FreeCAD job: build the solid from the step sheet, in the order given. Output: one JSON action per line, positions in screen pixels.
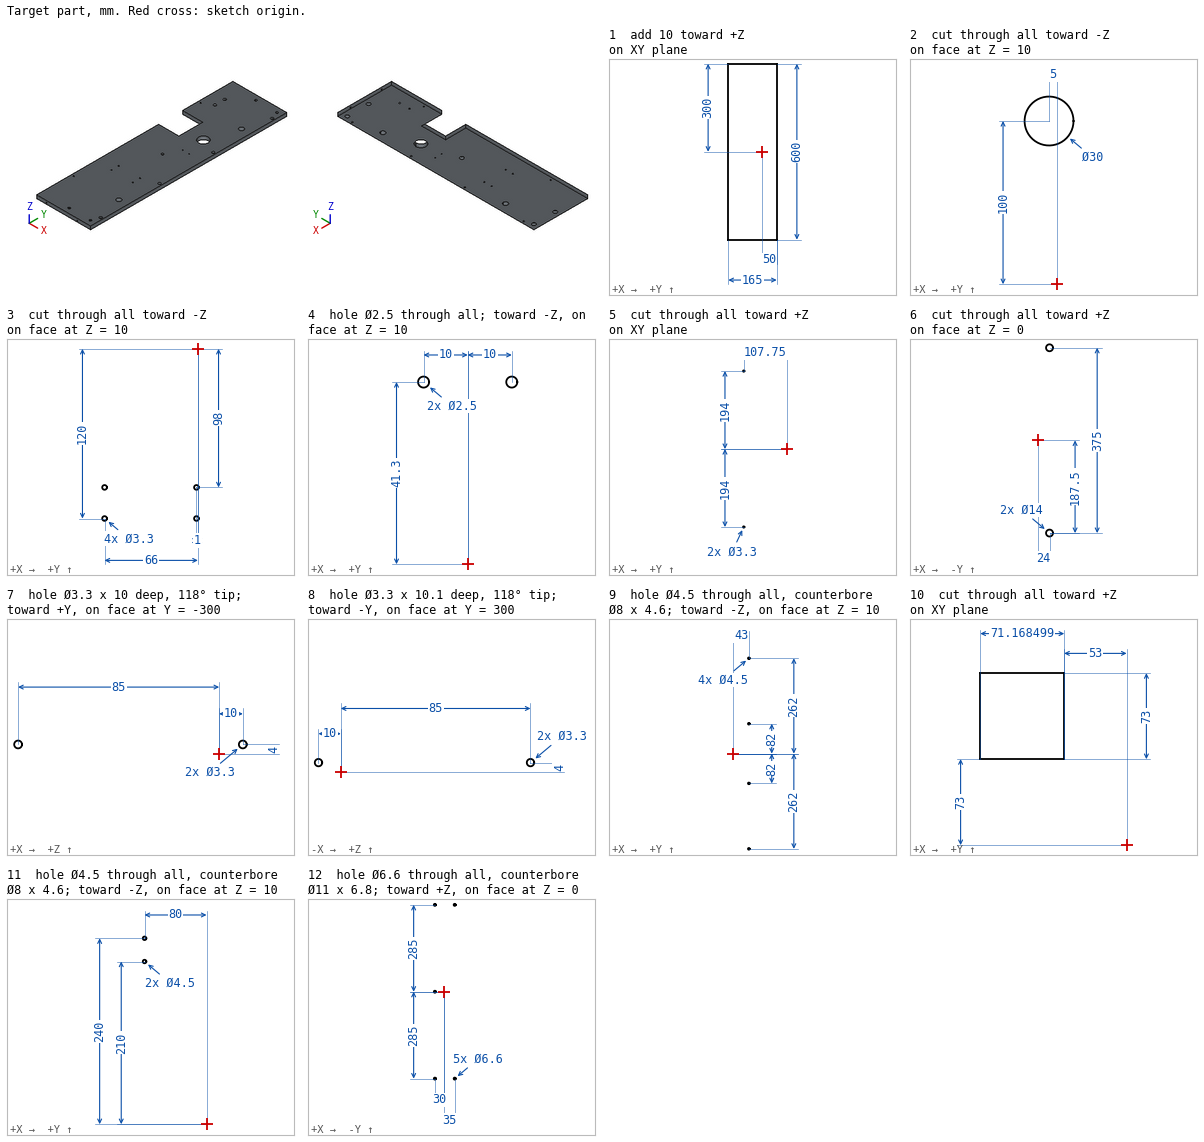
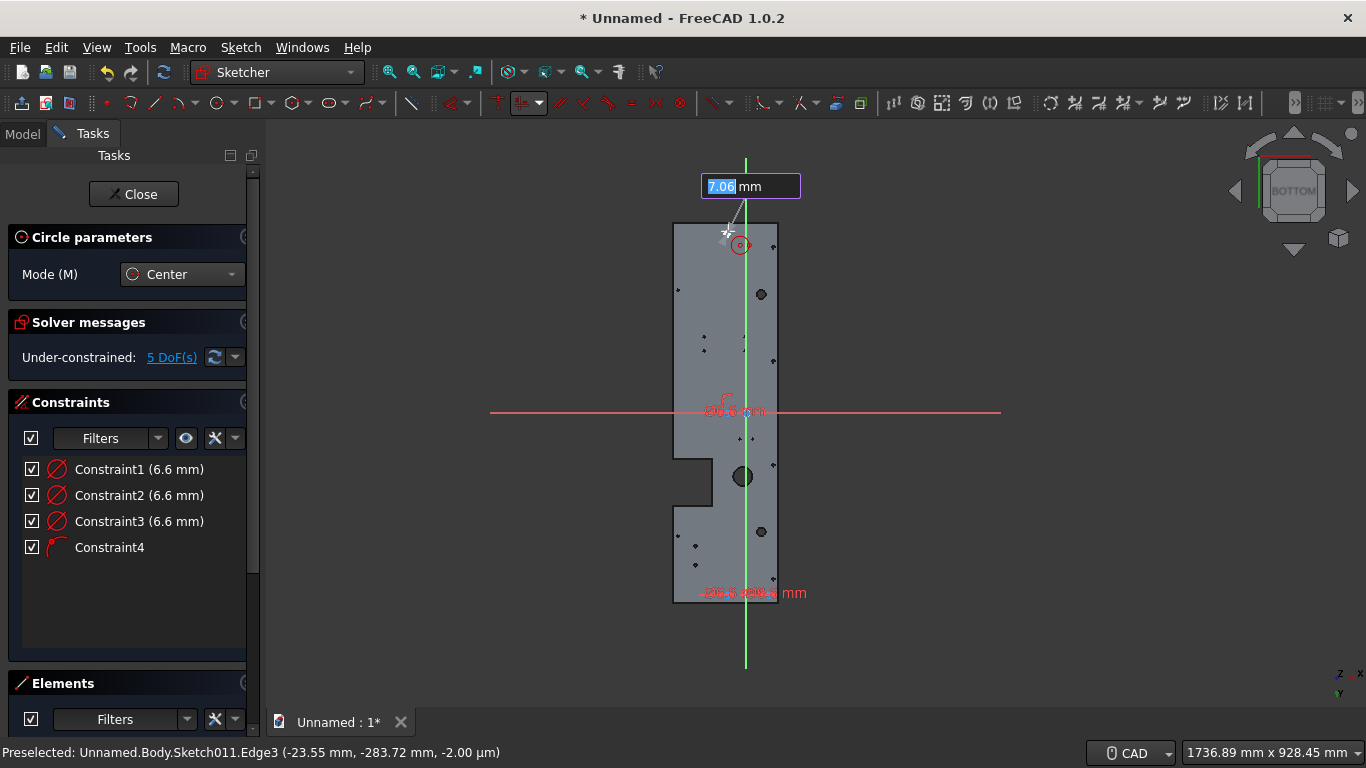
{"action": "type", "text": "6.6"}
{"action": "key", "text": "Return"}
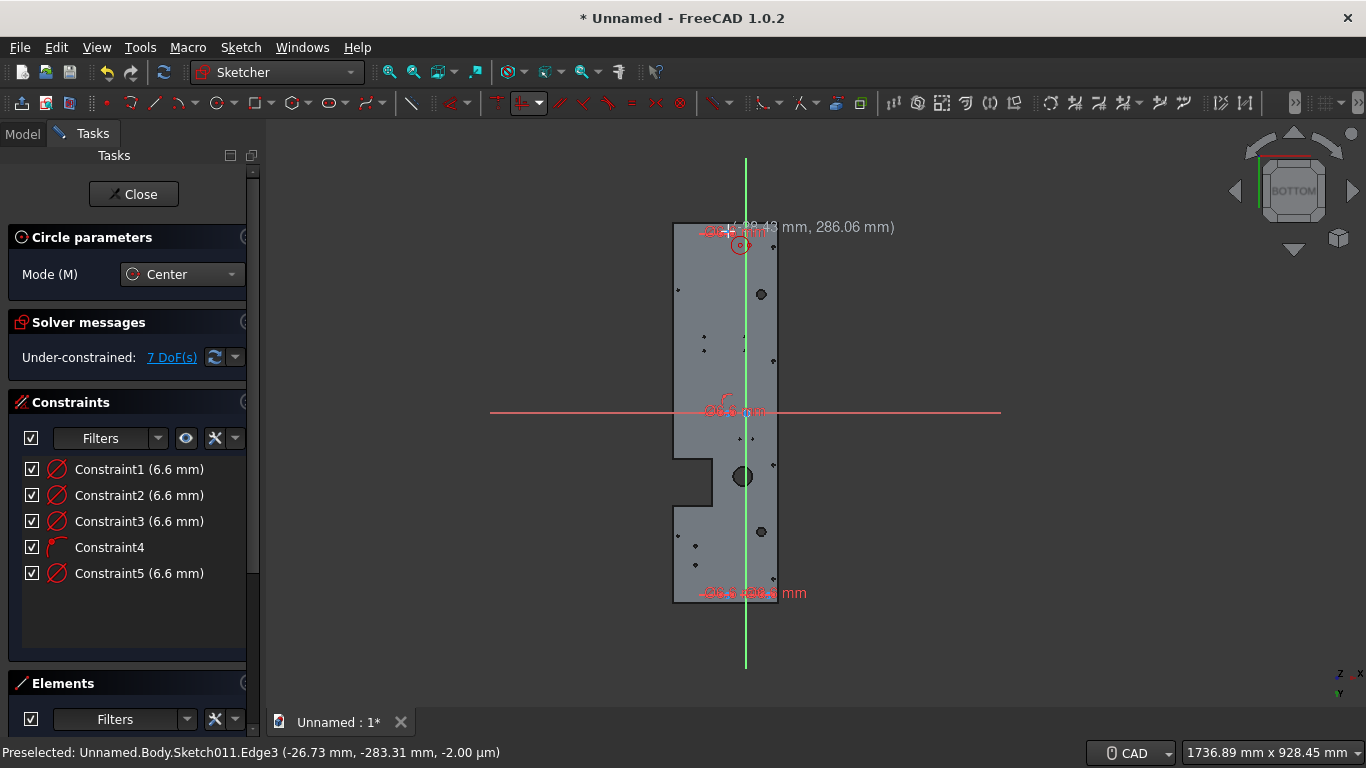
{"action": "scroll", "coordinate": [768, 233], "scroll_direction": "up", "scroll_amount": 12}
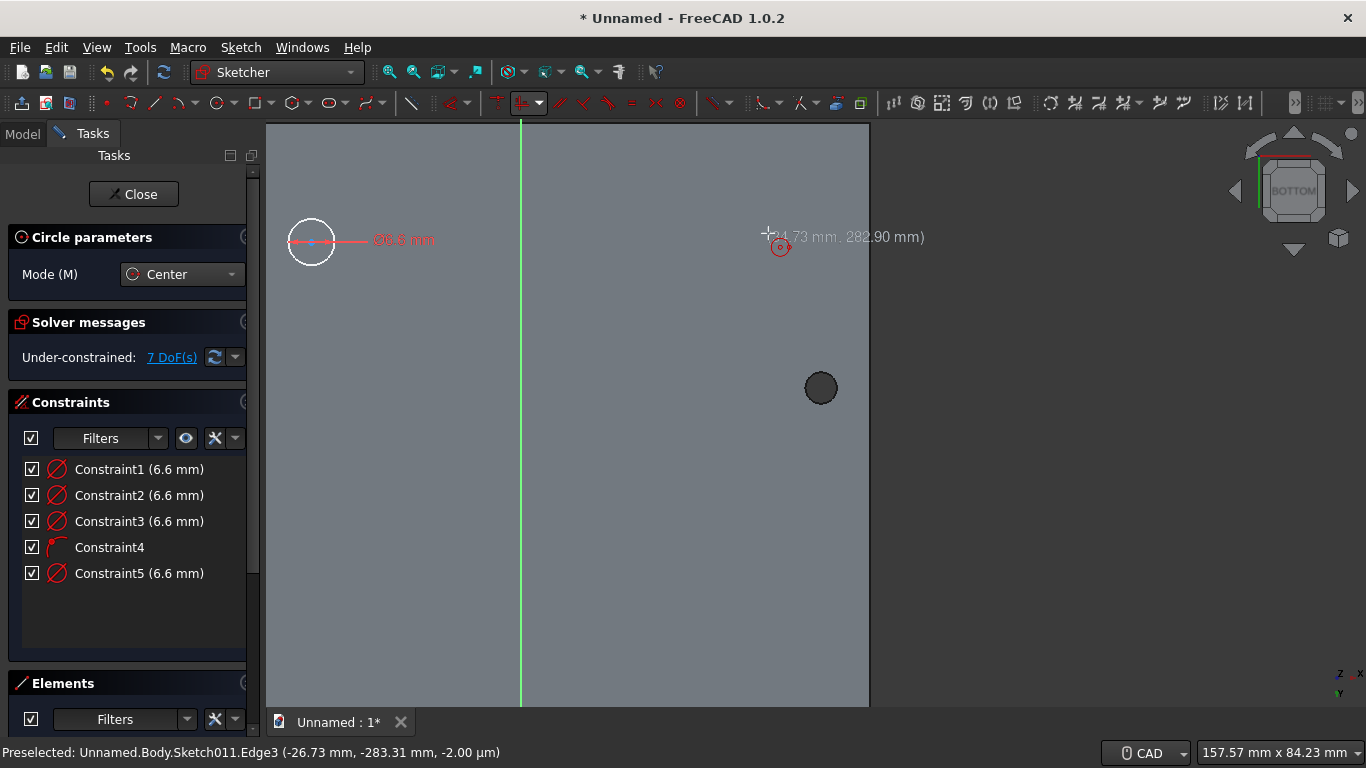
{"action": "scroll", "coordinate": [768, 233], "scroll_direction": "down", "scroll_amount": 12}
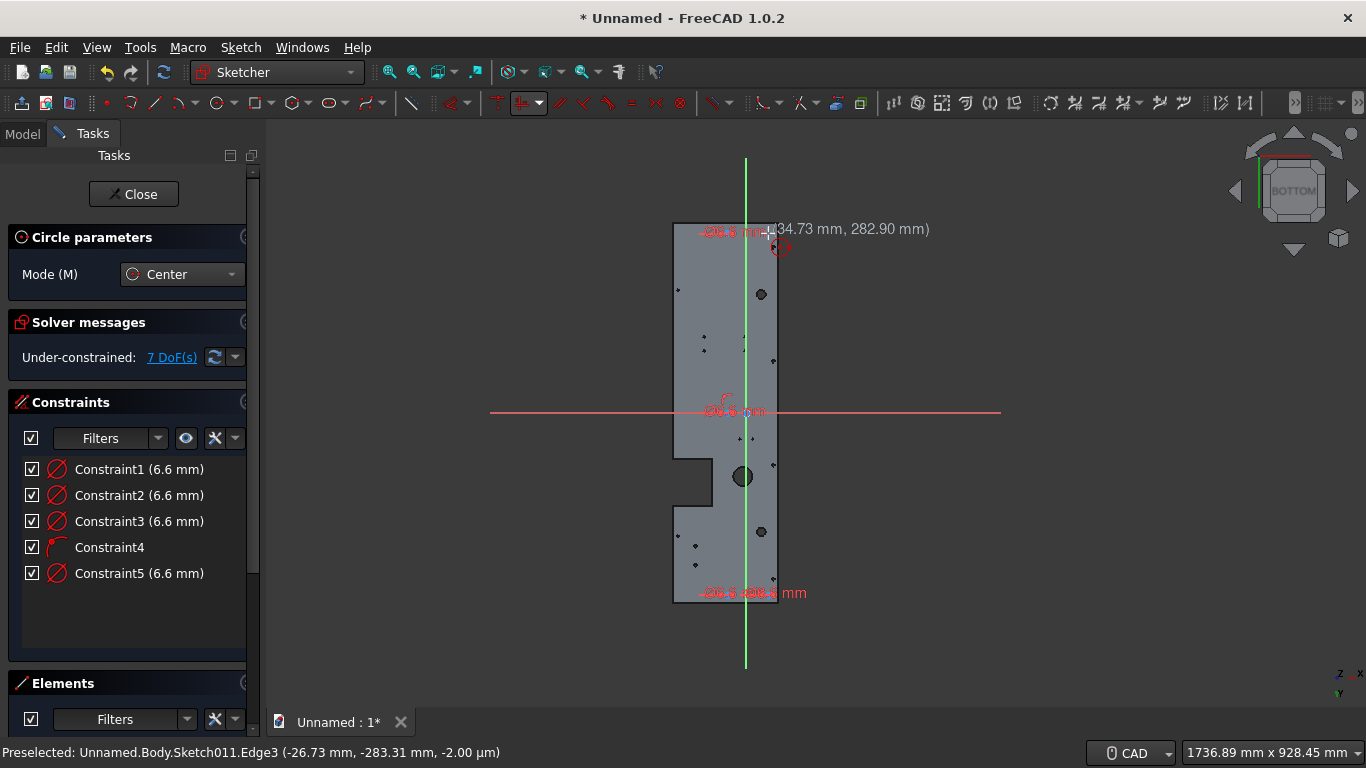
{"action": "left_click", "coordinate": [768, 233]}
{"action": "mouse_move", "coordinate": [770, 231]}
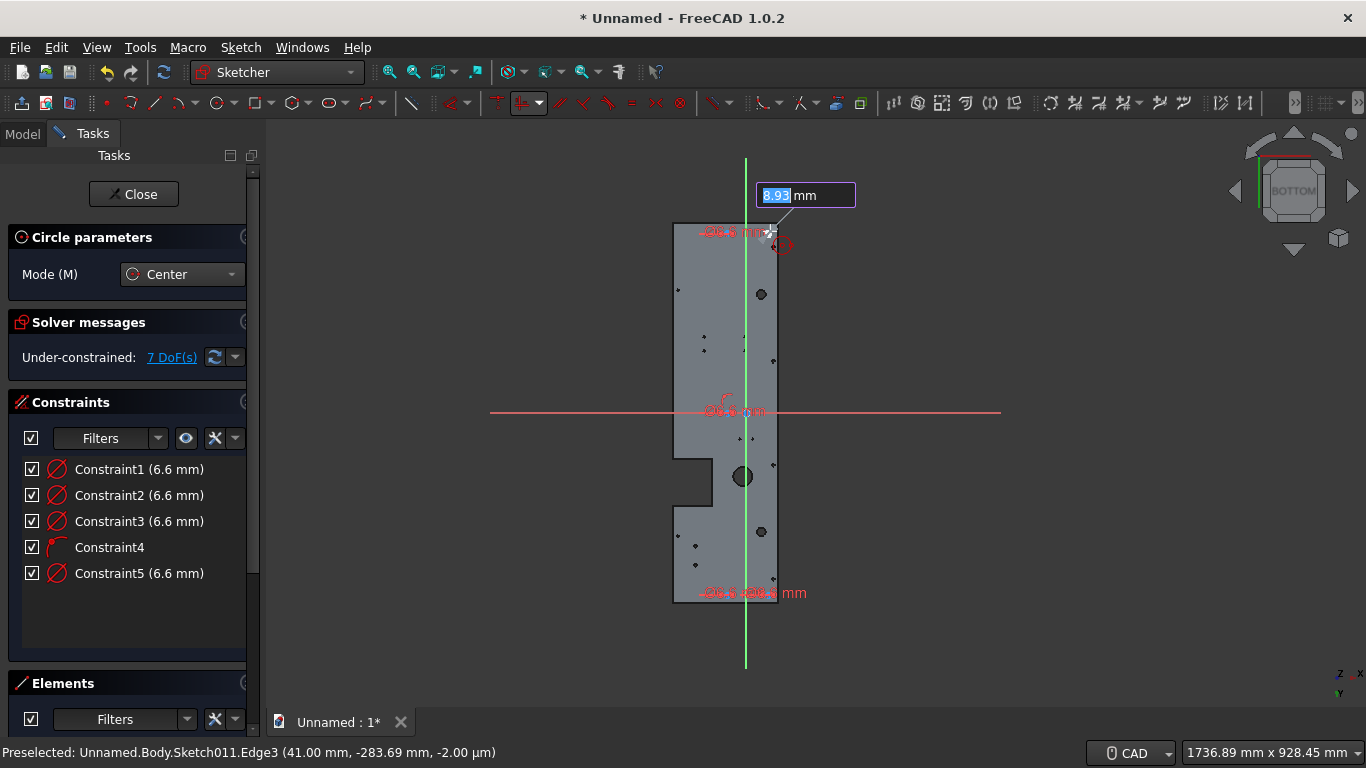
{"action": "type", "text": "6.6"}
{"action": "key", "text": "Return"}
{"action": "key", "text": "Escape"}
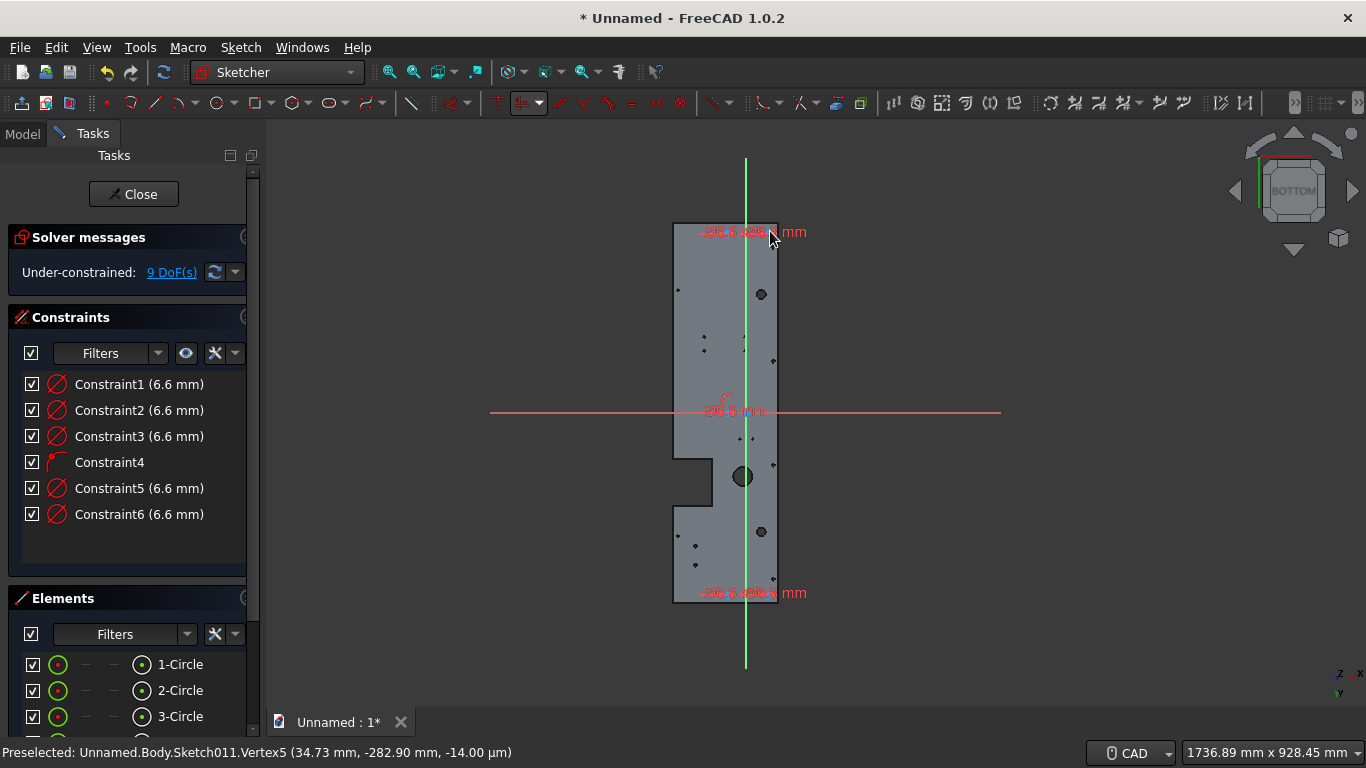
{"action": "left_click", "coordinate": [727, 595]}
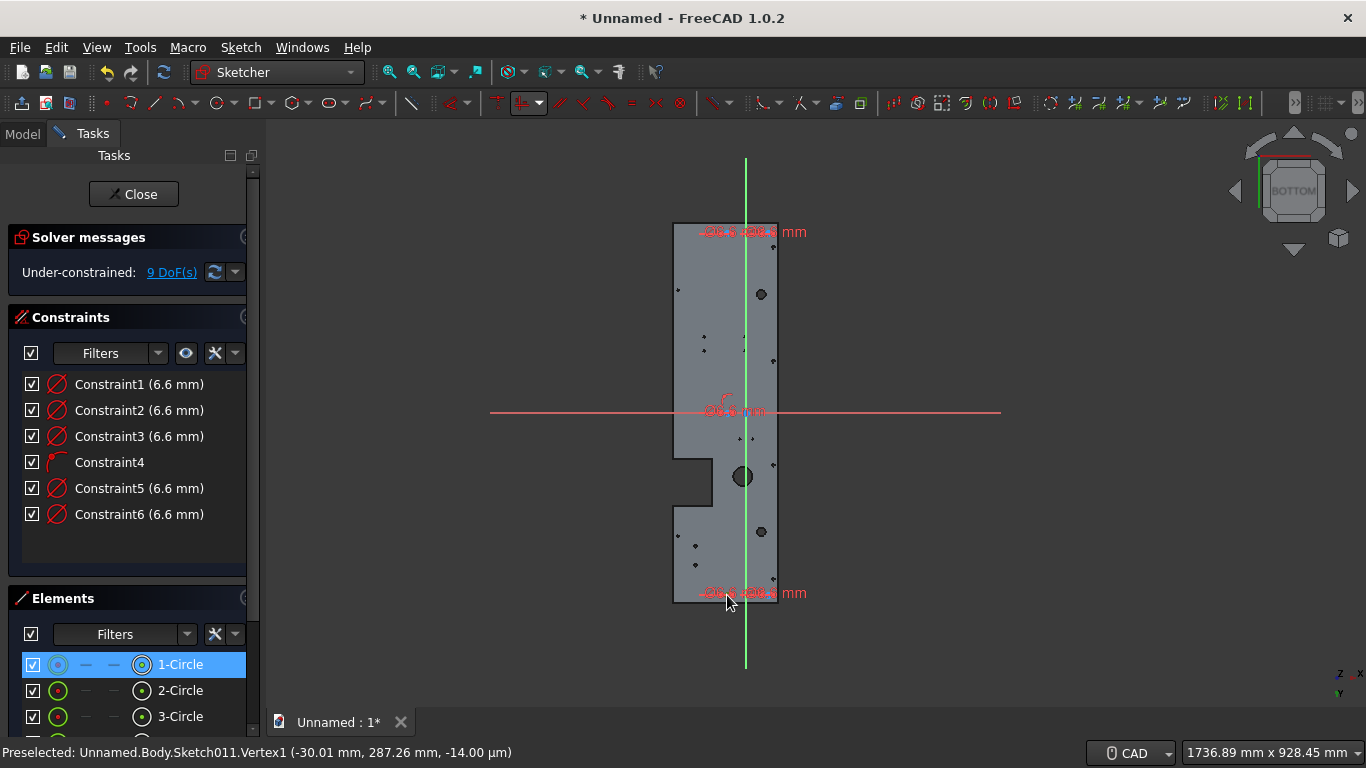
{"action": "left_click", "coordinate": [768, 595]}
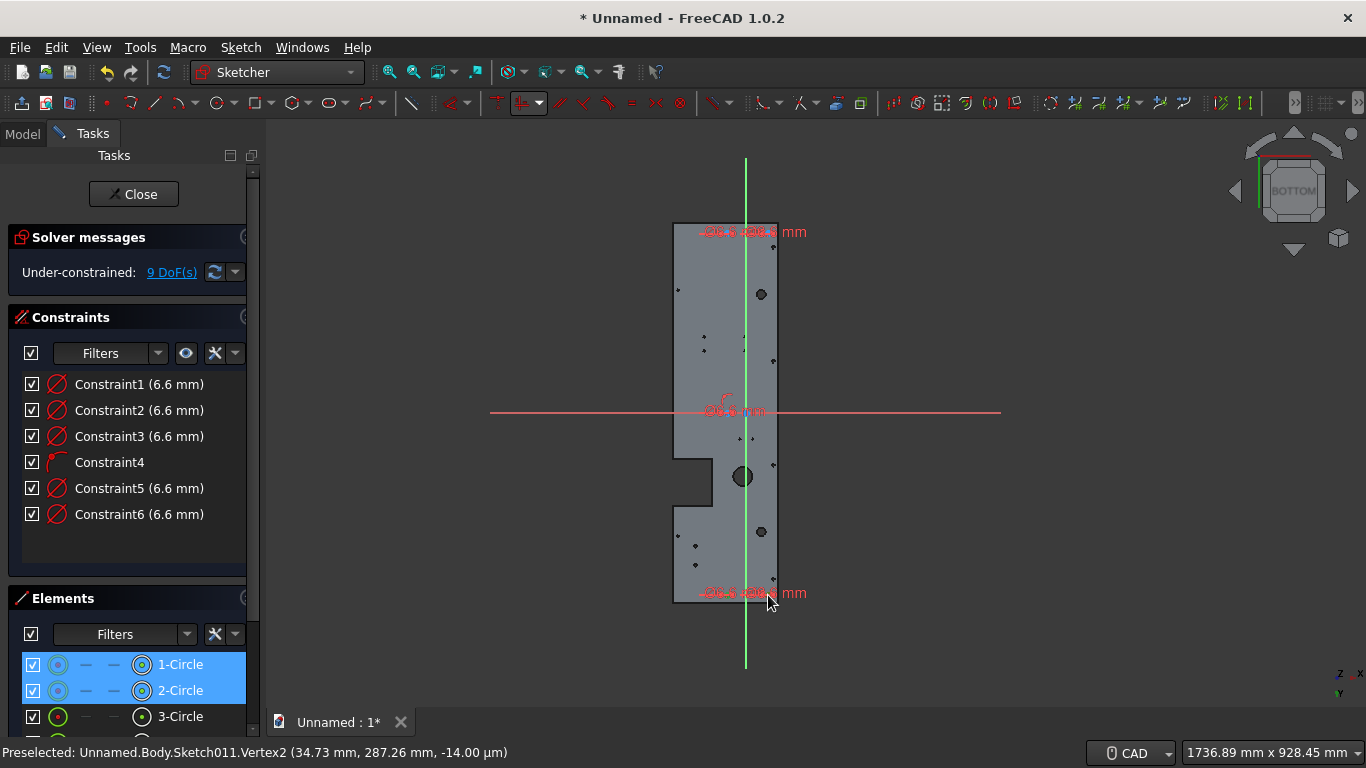
{"action": "left_click", "coordinate": [542, 104]}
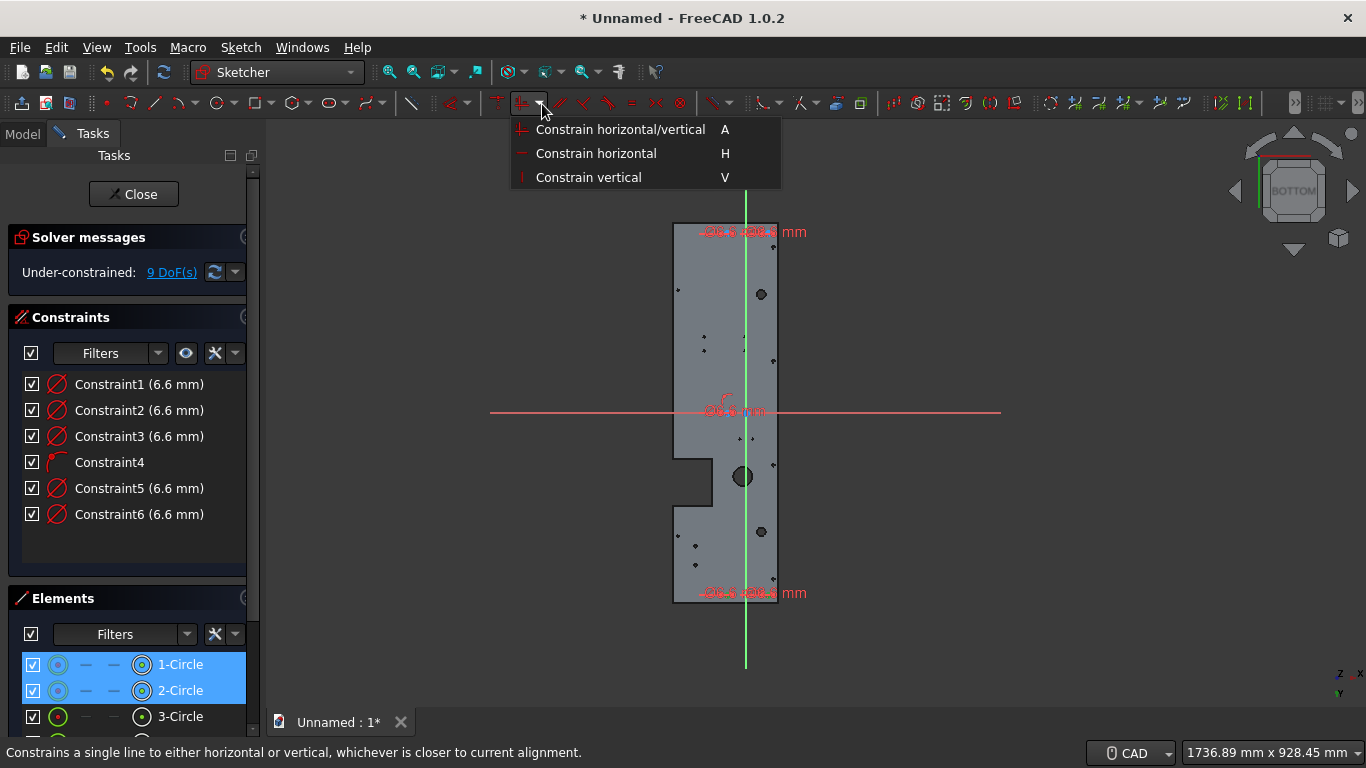
{"action": "left_click", "coordinate": [646, 153]}